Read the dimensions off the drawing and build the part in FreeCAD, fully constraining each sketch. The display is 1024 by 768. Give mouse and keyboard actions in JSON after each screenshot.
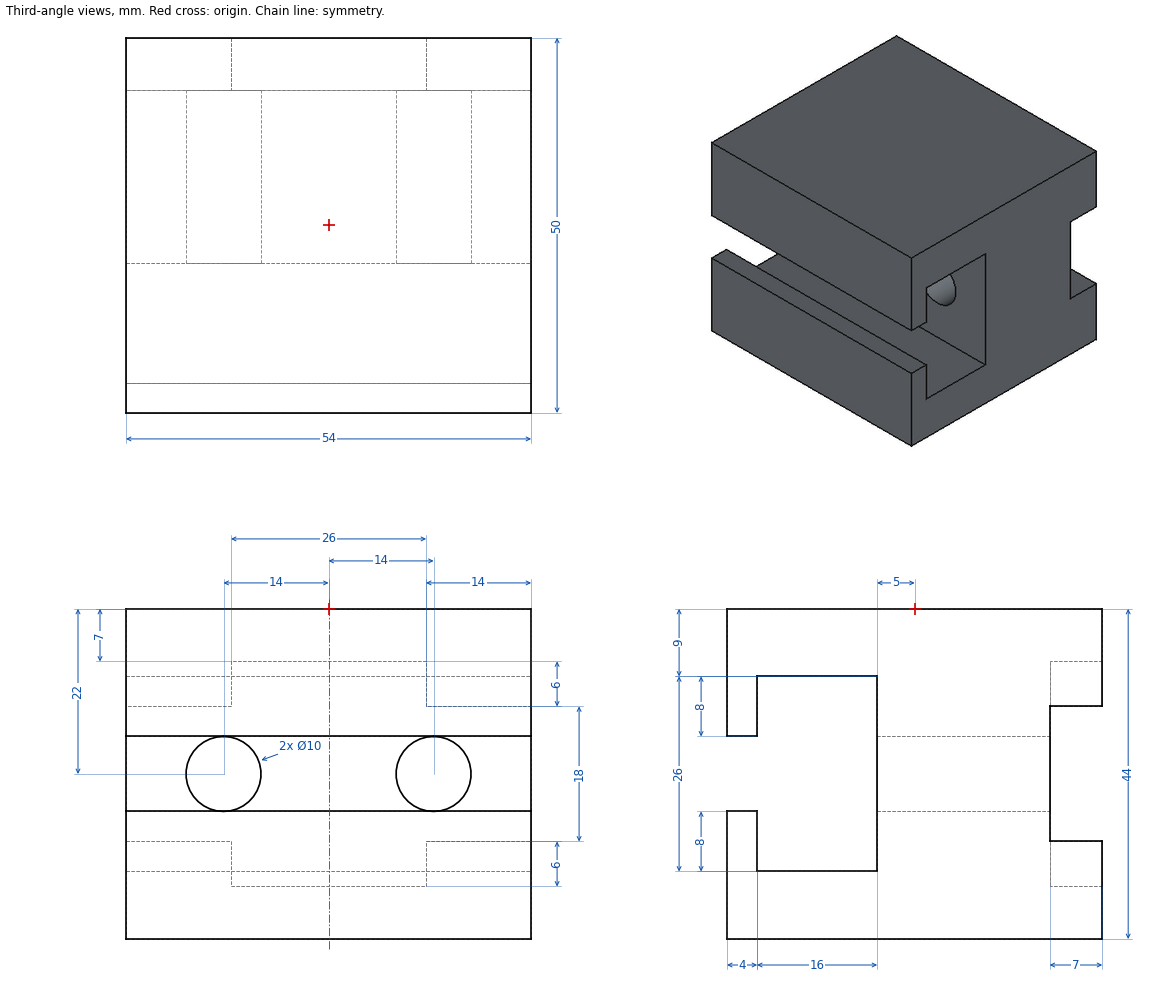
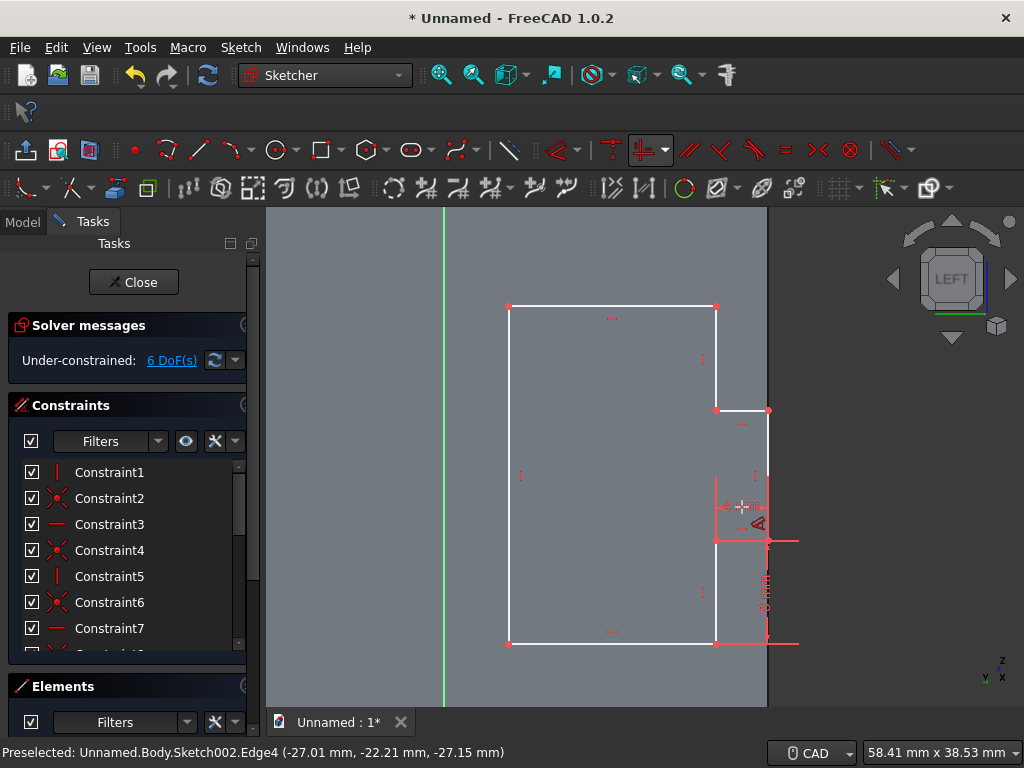
{"action": "left_click", "coordinate": [753, 411]}
{"action": "left_click", "coordinate": [742, 377]}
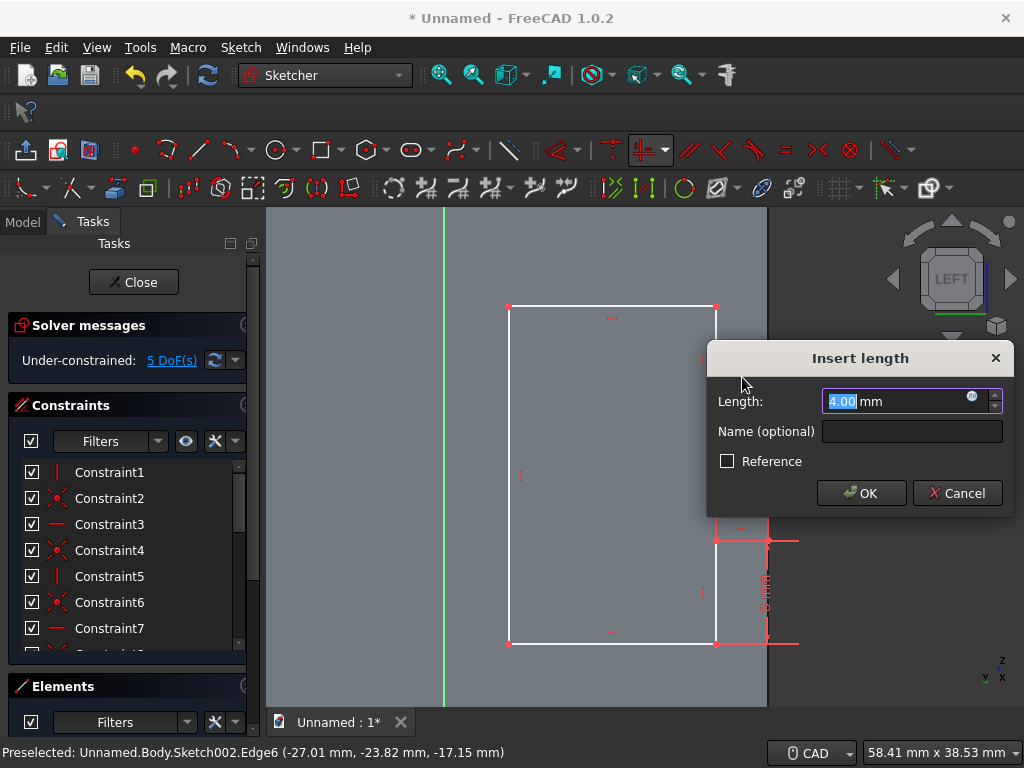
{"action": "type", "text": "4"}
{"action": "key", "text": "Return"}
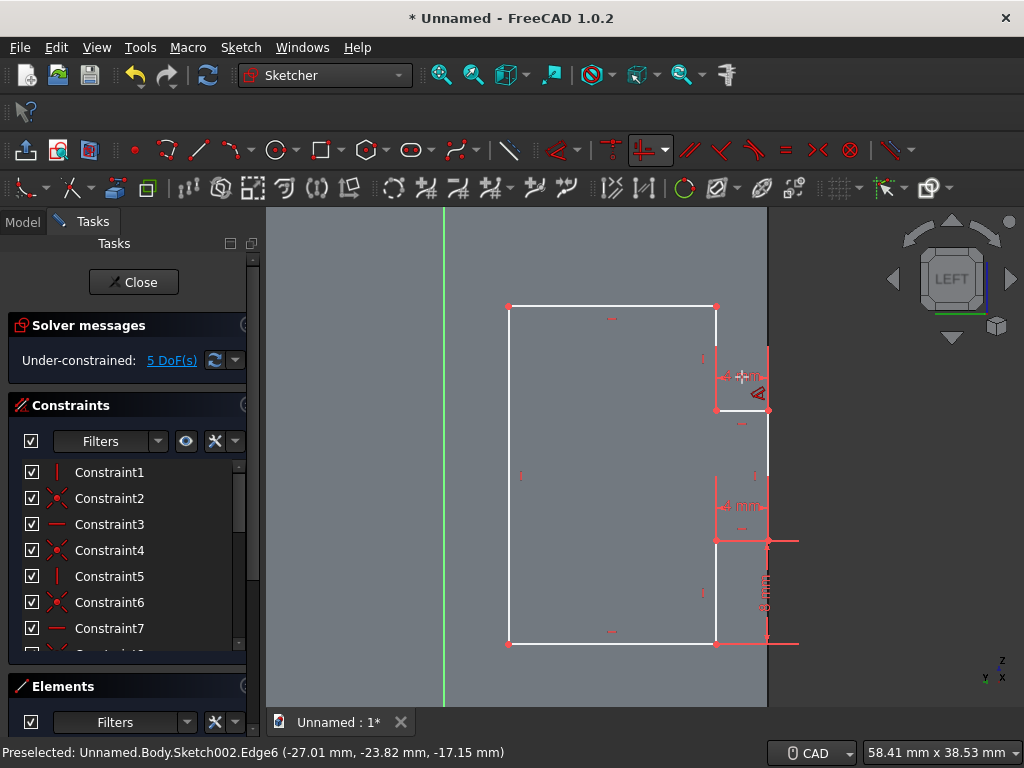
{"action": "left_click", "coordinate": [716, 380]}
{"action": "left_click", "coordinate": [750, 335]}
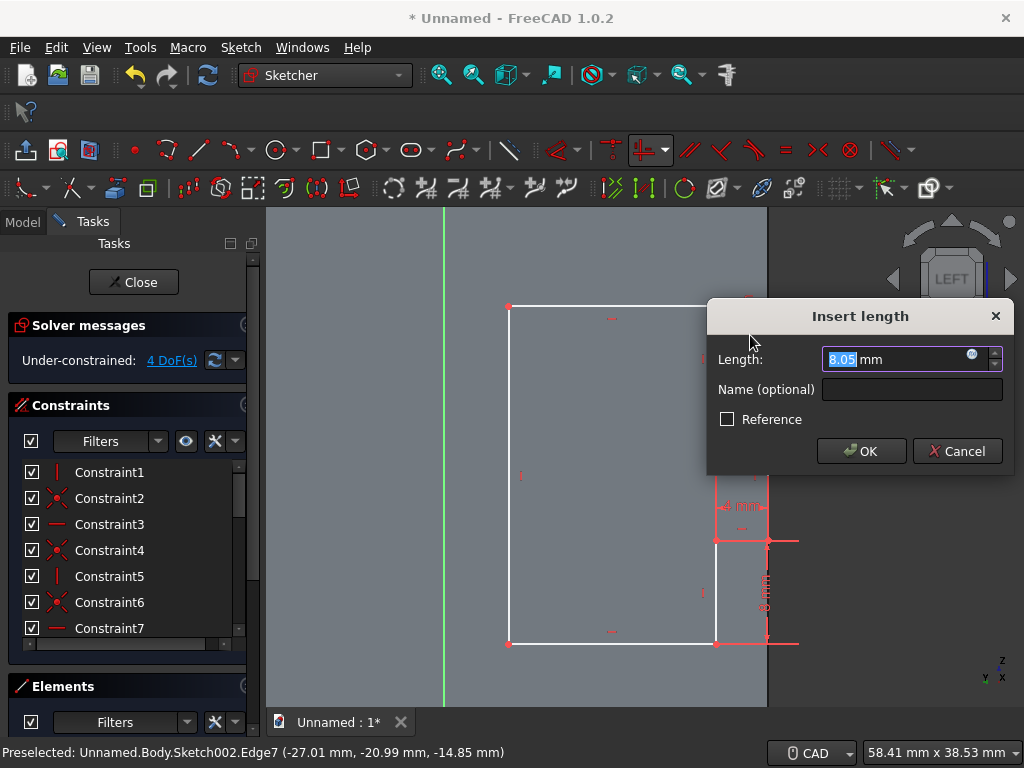
{"action": "type", "text": "8"}
{"action": "key", "text": "Return"}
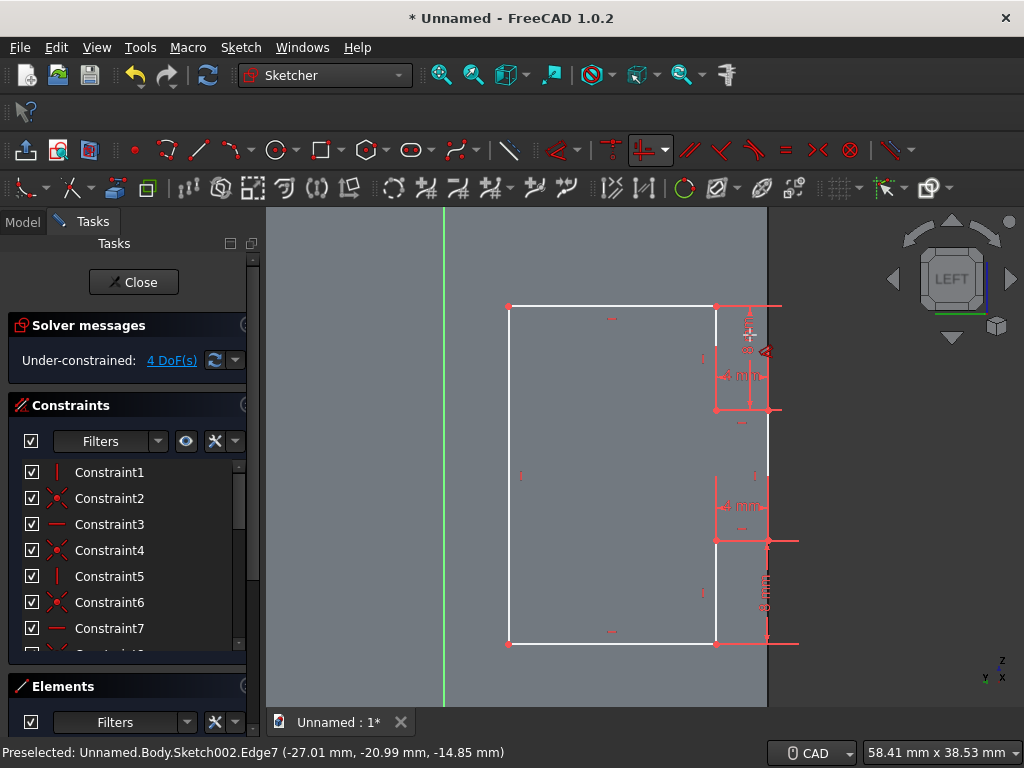
{"action": "left_click", "coordinate": [509, 408]}
{"action": "left_click", "coordinate": [475, 475]}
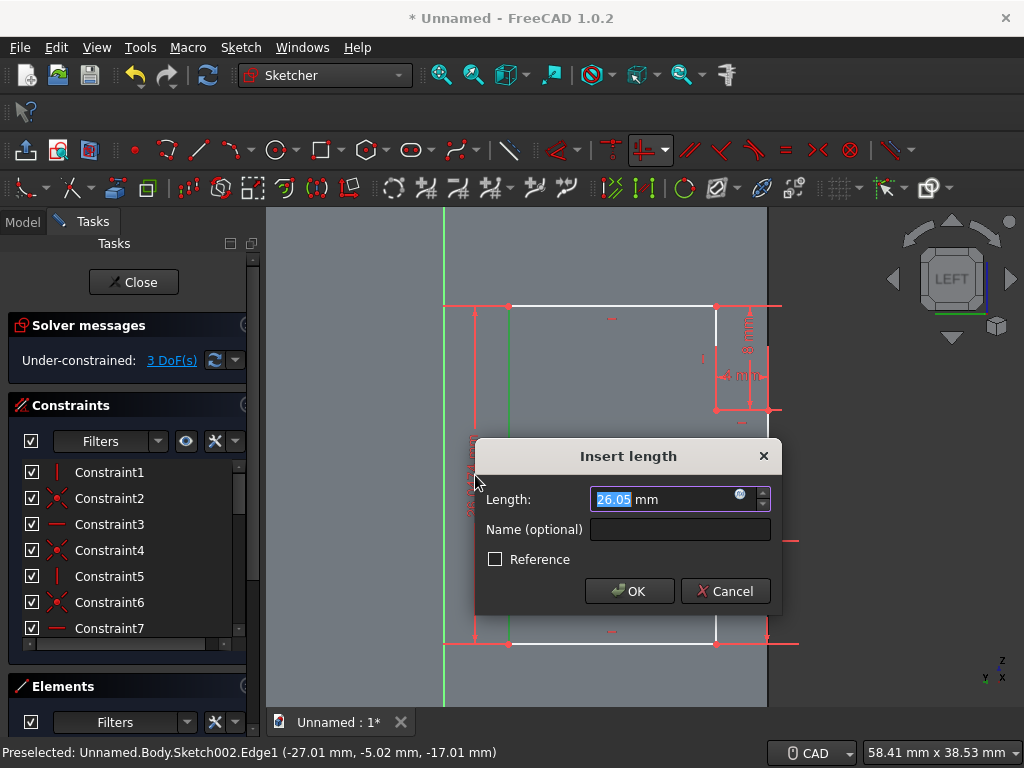
{"action": "type", "text": "26"}
{"action": "key", "text": "Return"}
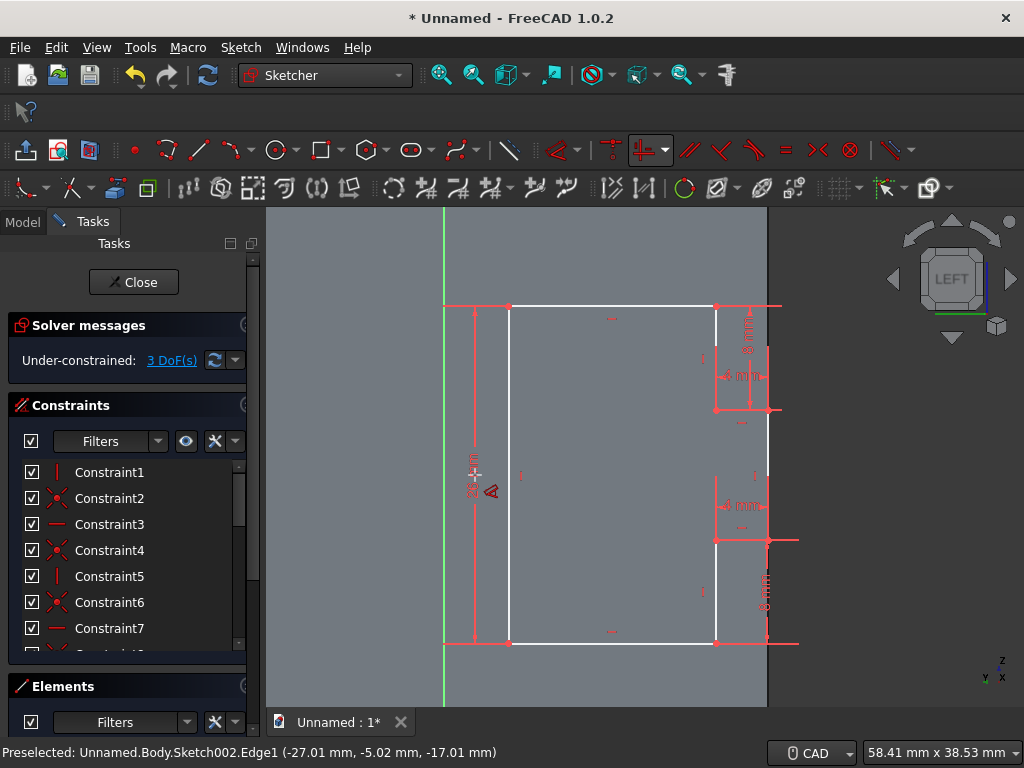
{"action": "left_click", "coordinate": [571, 644]}
{"action": "left_click", "coordinate": [613, 678]}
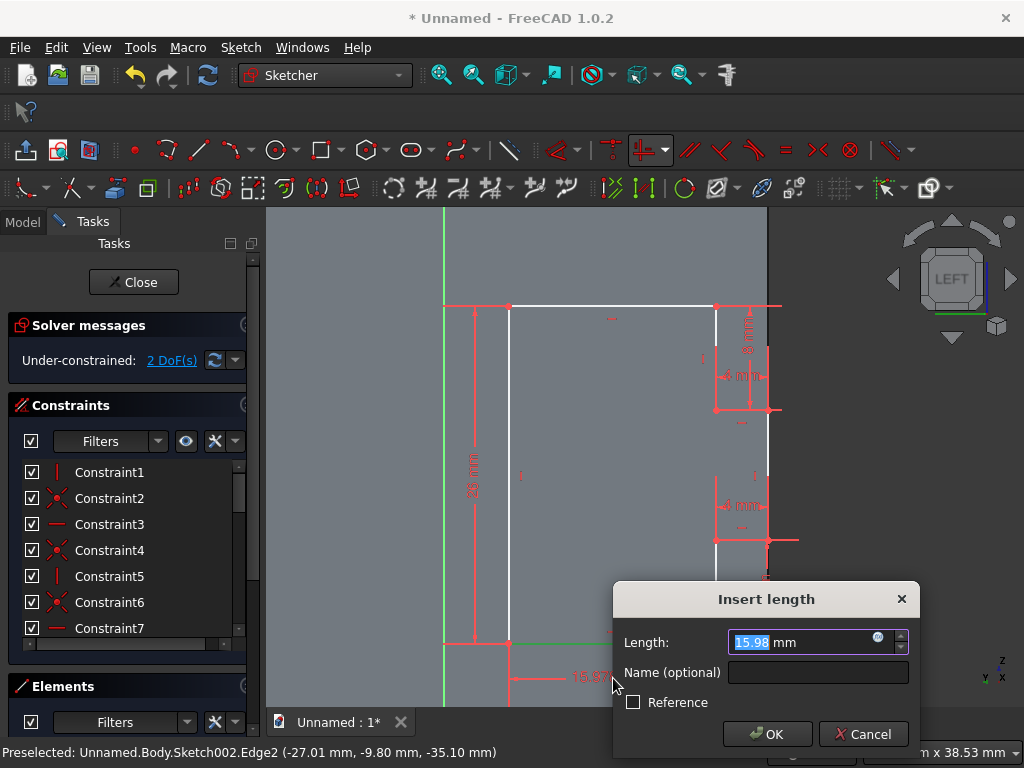
{"action": "type", "text": "16"}
{"action": "key", "text": "Return"}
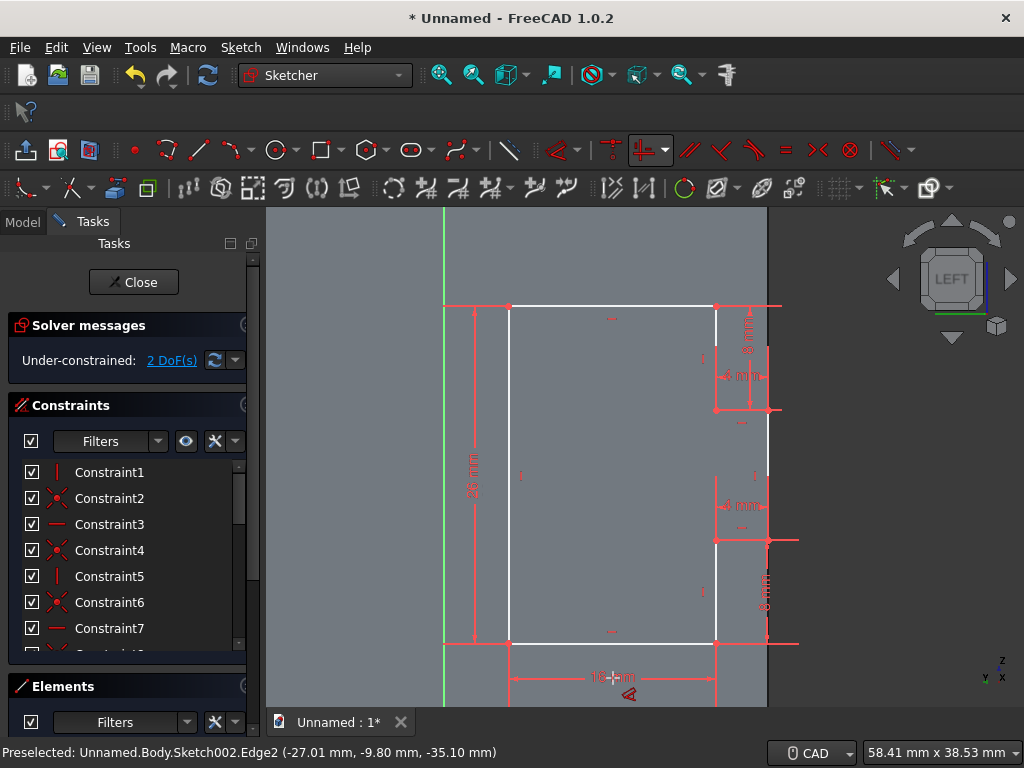
{"action": "left_click", "coordinate": [509, 306]}
{"action": "left_click", "coordinate": [476, 340]}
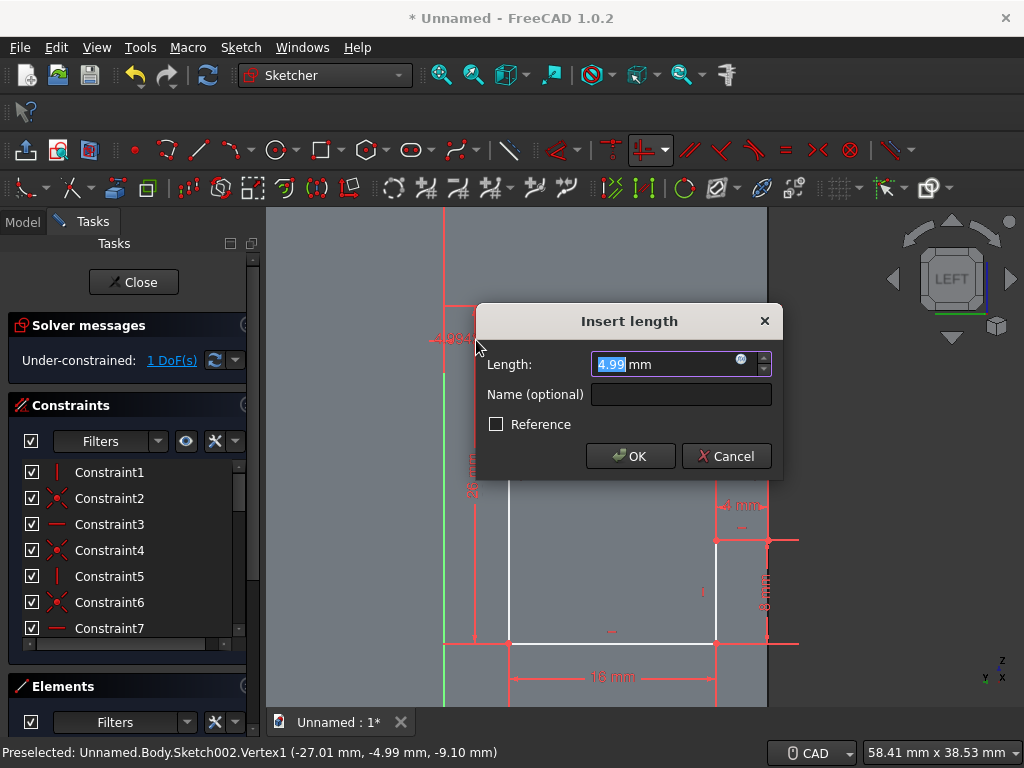
{"action": "type", "text": "5"}
{"action": "key", "text": "Return"}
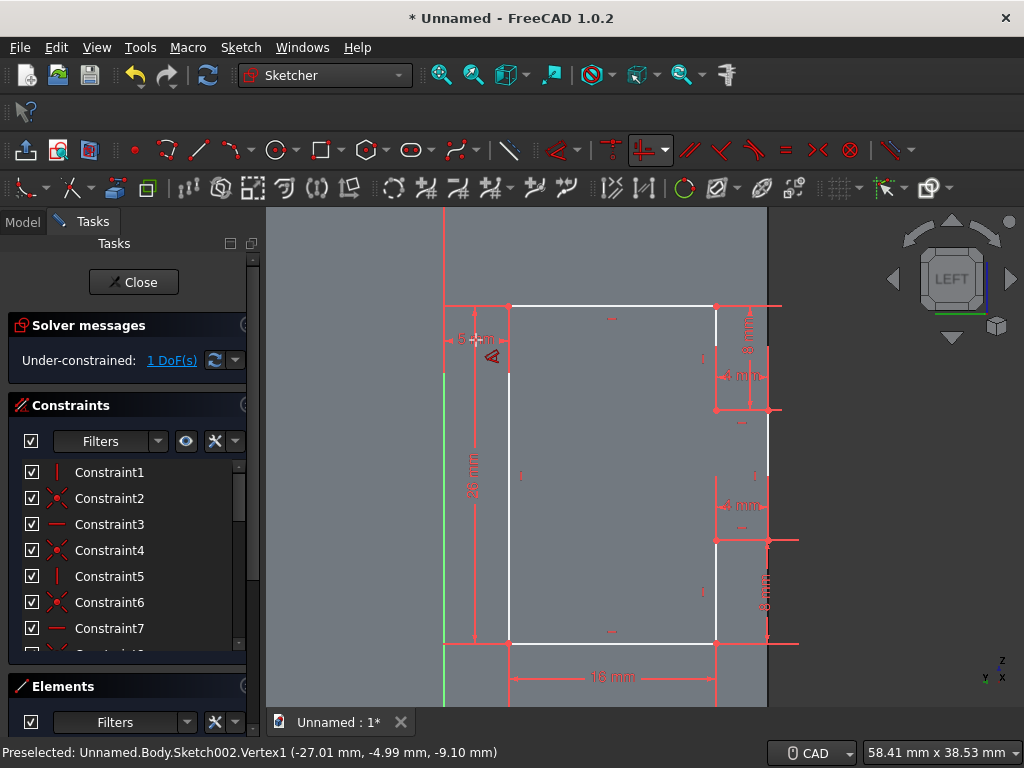
{"action": "left_click", "coordinate": [509, 306]}
{"action": "left_click", "coordinate": [410, 271]}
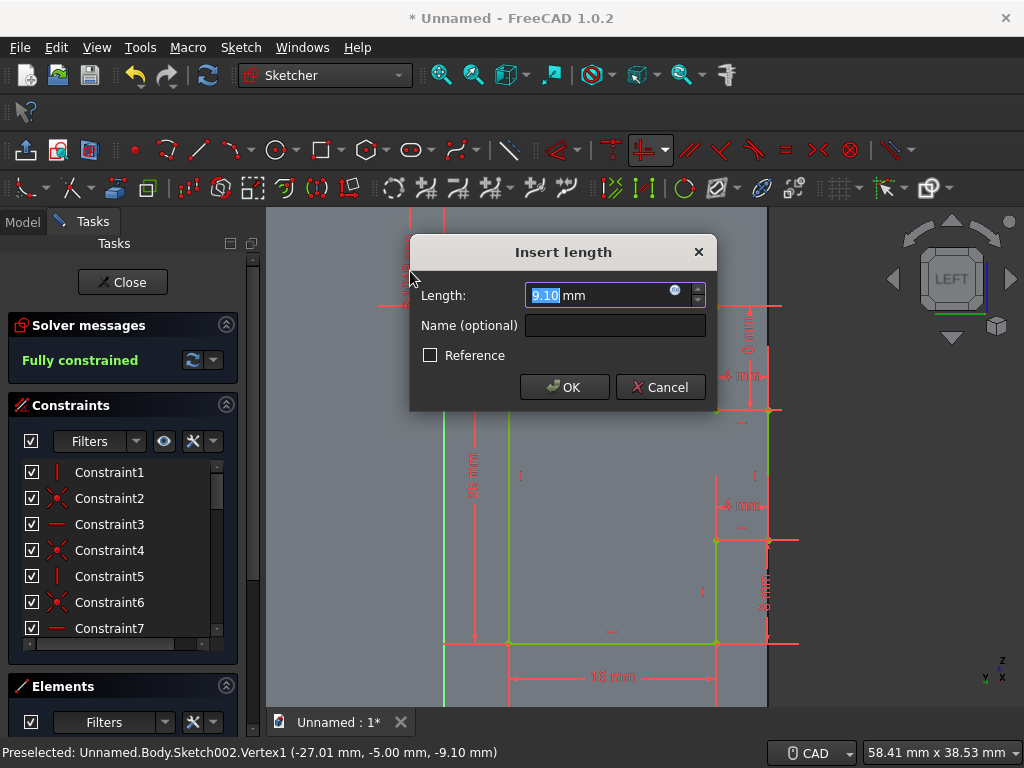
{"action": "type", "text": "9"}
{"action": "key", "text": "Return"}
{"action": "key", "text": "Escape"}